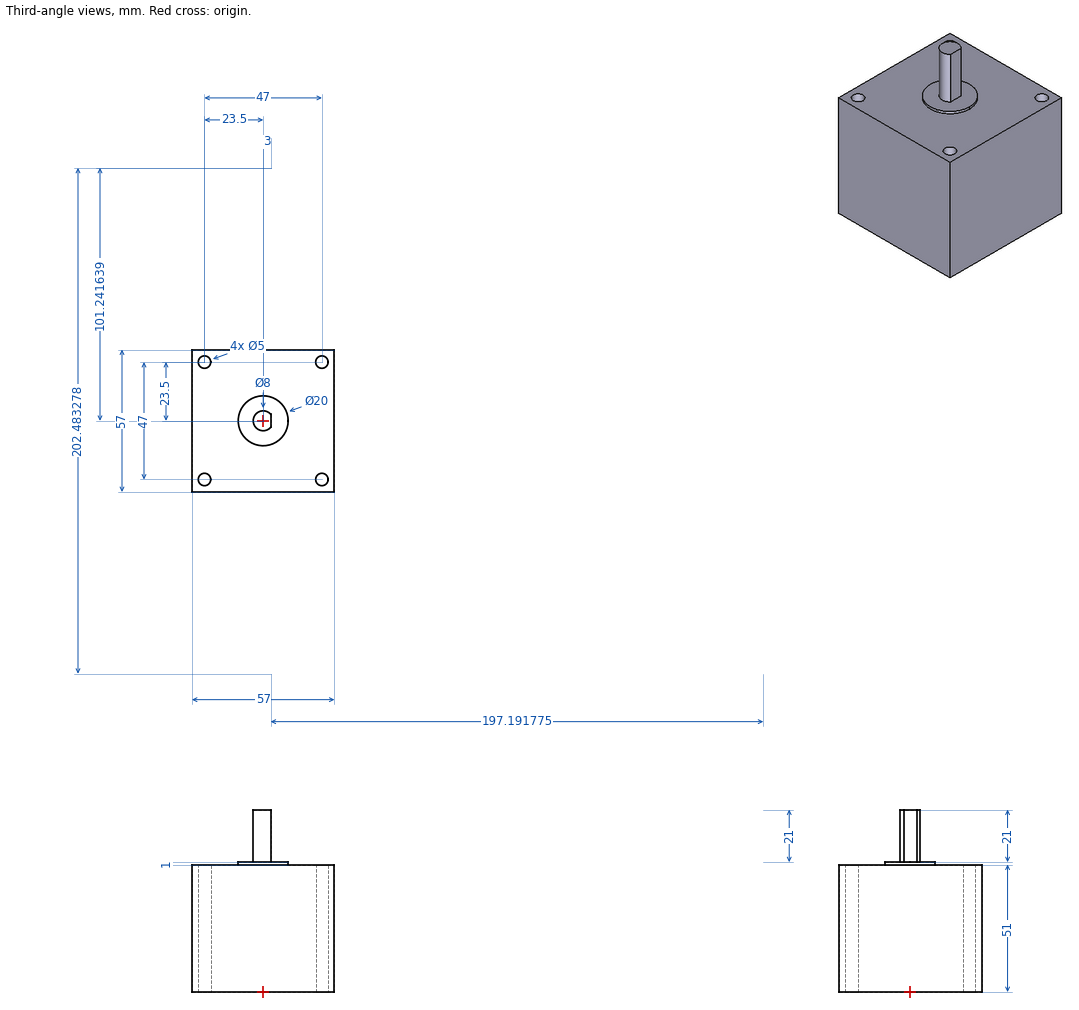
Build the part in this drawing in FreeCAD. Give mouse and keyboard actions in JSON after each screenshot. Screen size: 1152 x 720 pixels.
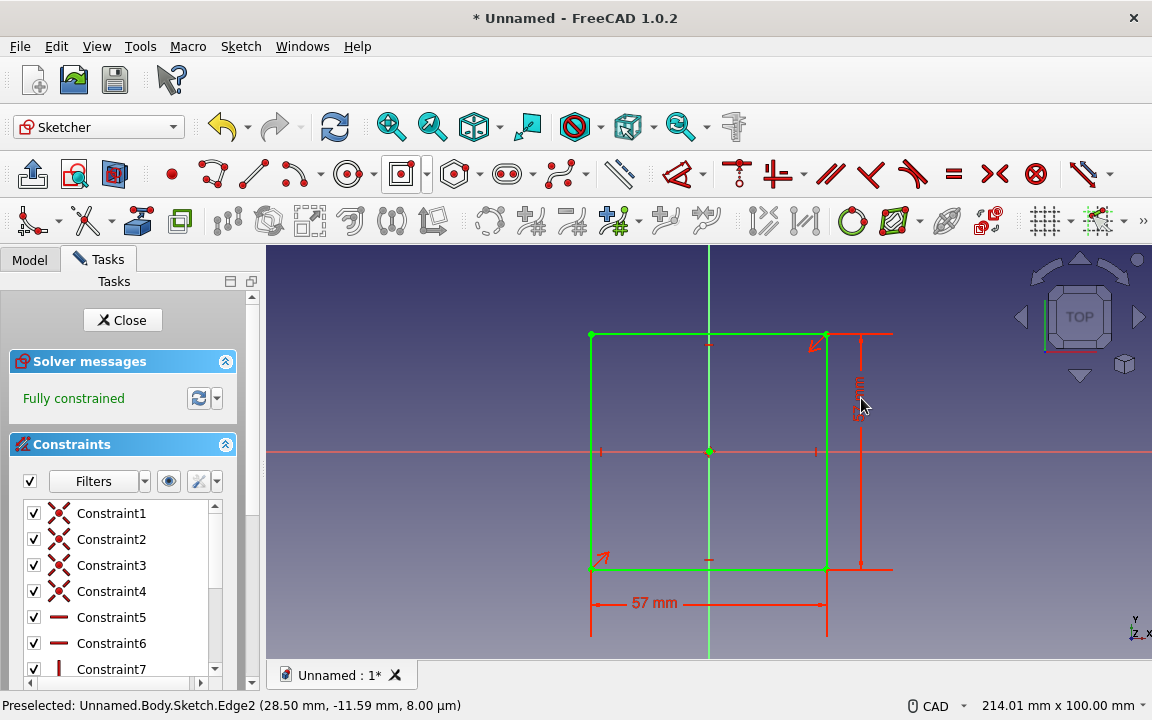
{"action": "left_click", "coordinate": [123, 320]}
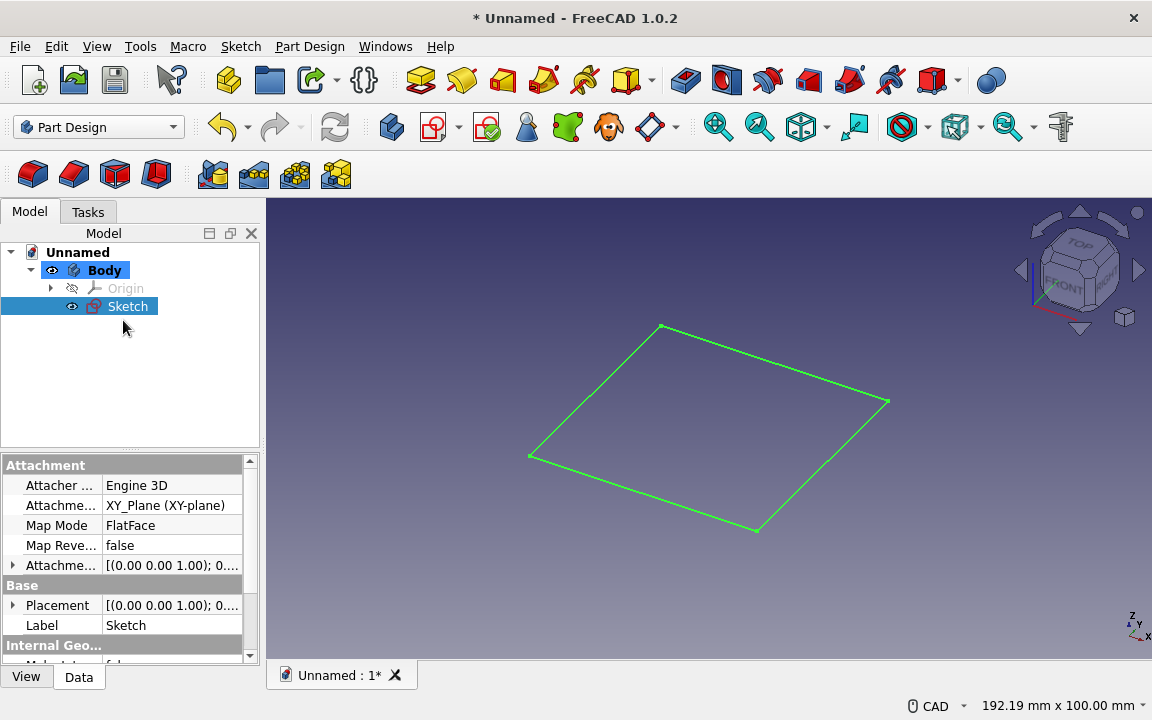
{"action": "left_click", "coordinate": [421, 80]}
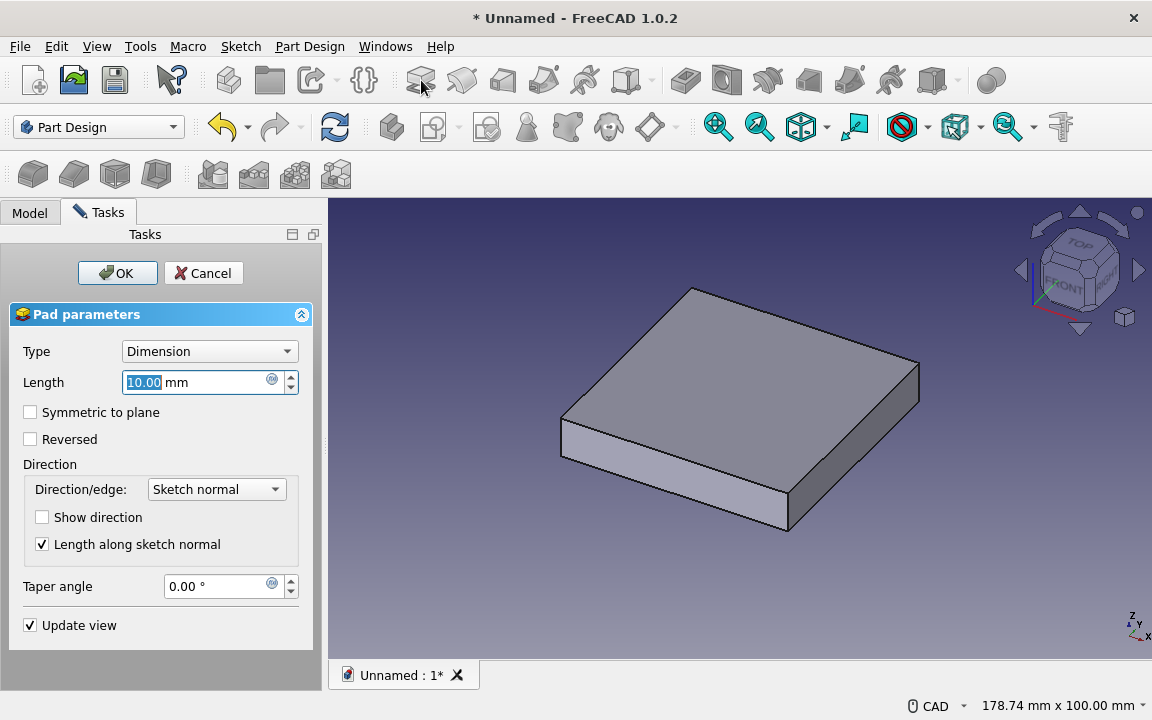
{"action": "type", "text": "51"}
{"action": "key", "text": "Tab"}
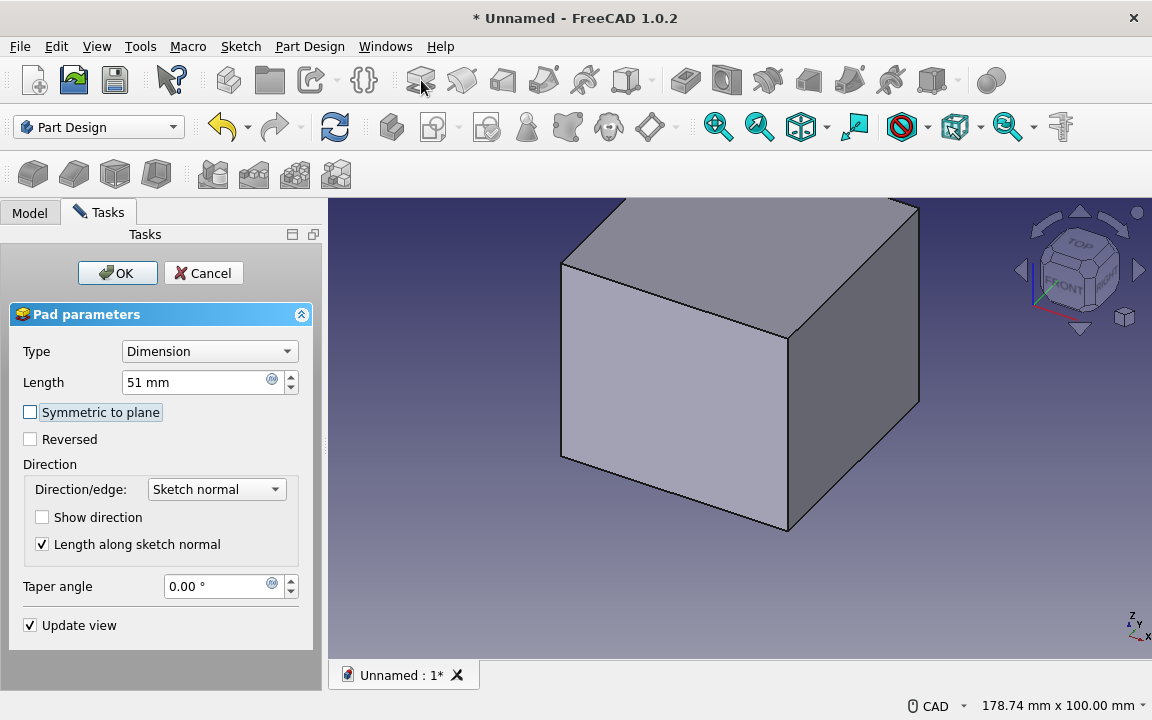
{"action": "left_click", "coordinate": [118, 273]}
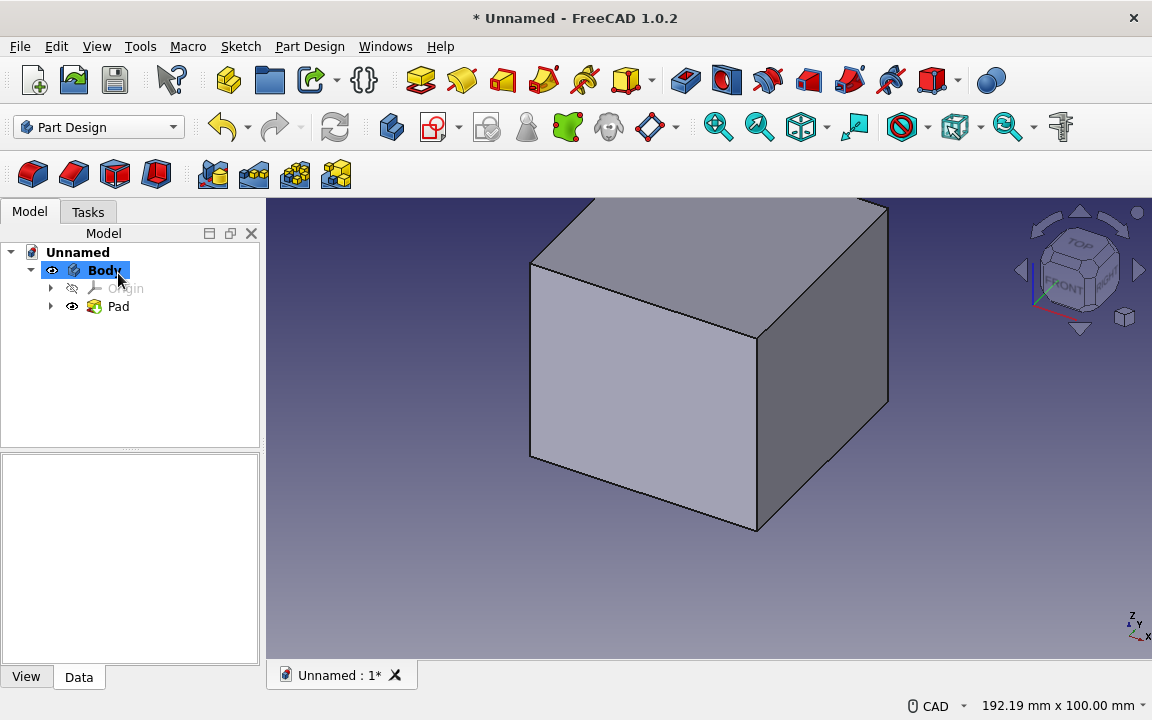
{"action": "left_click", "coordinate": [719, 128]}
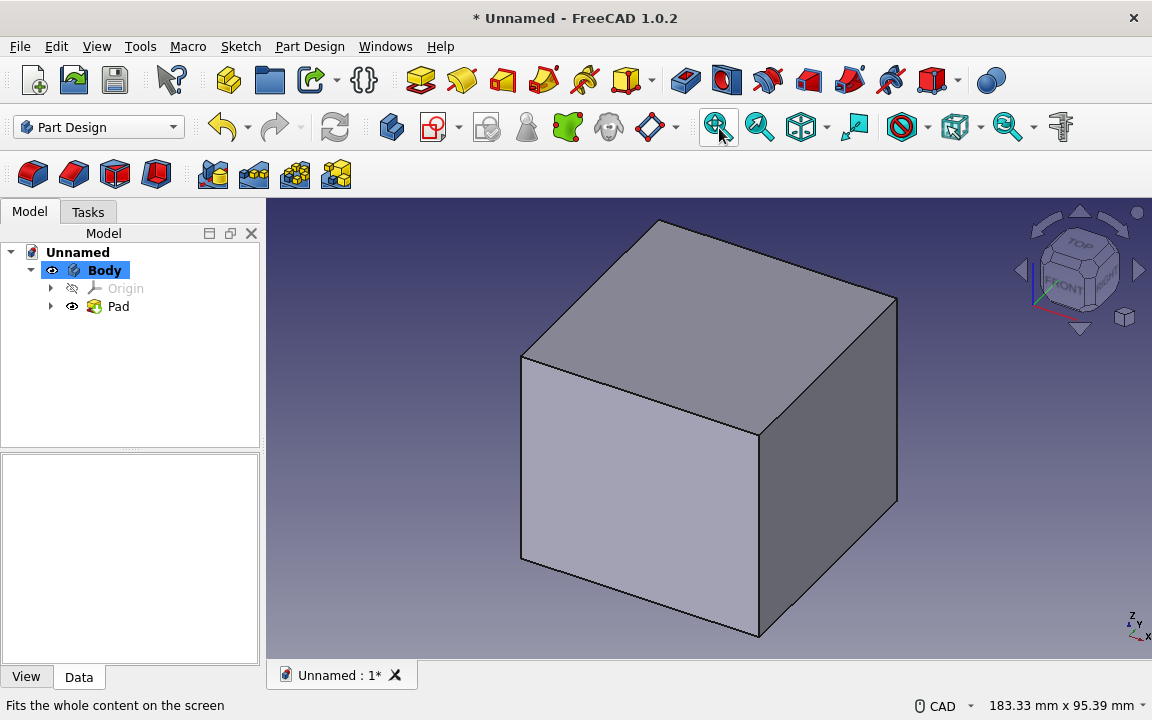
{"action": "left_click", "coordinate": [709, 327]}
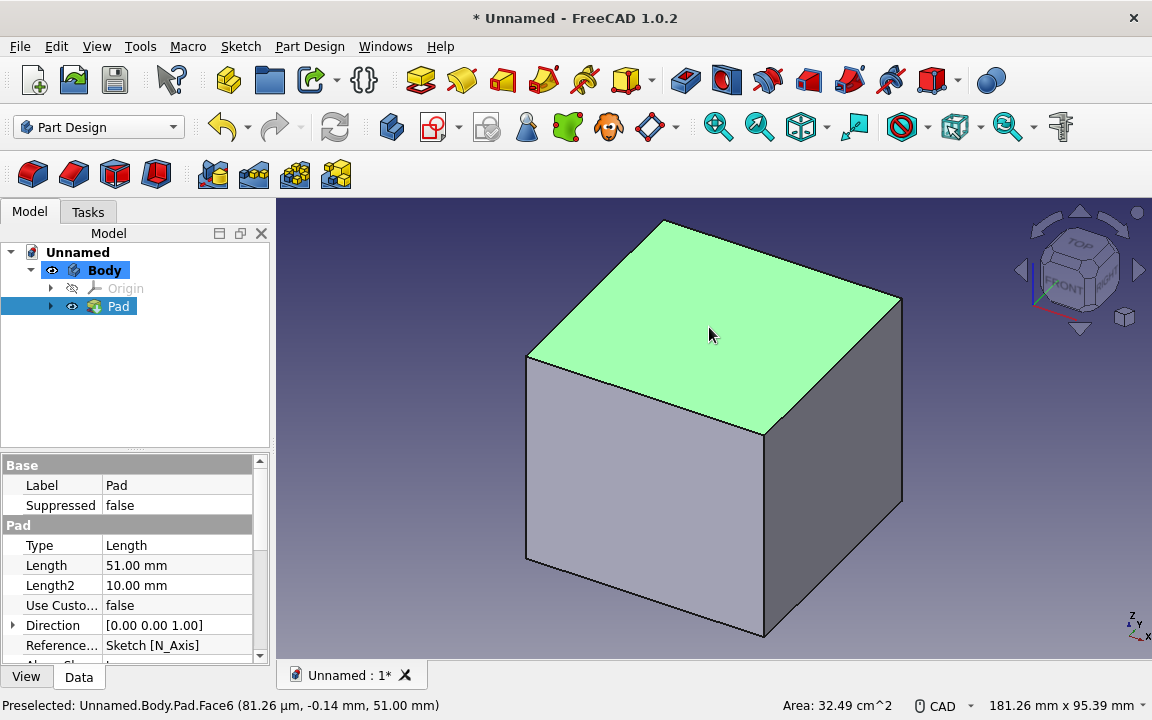
{"action": "left_click", "coordinate": [432, 128]}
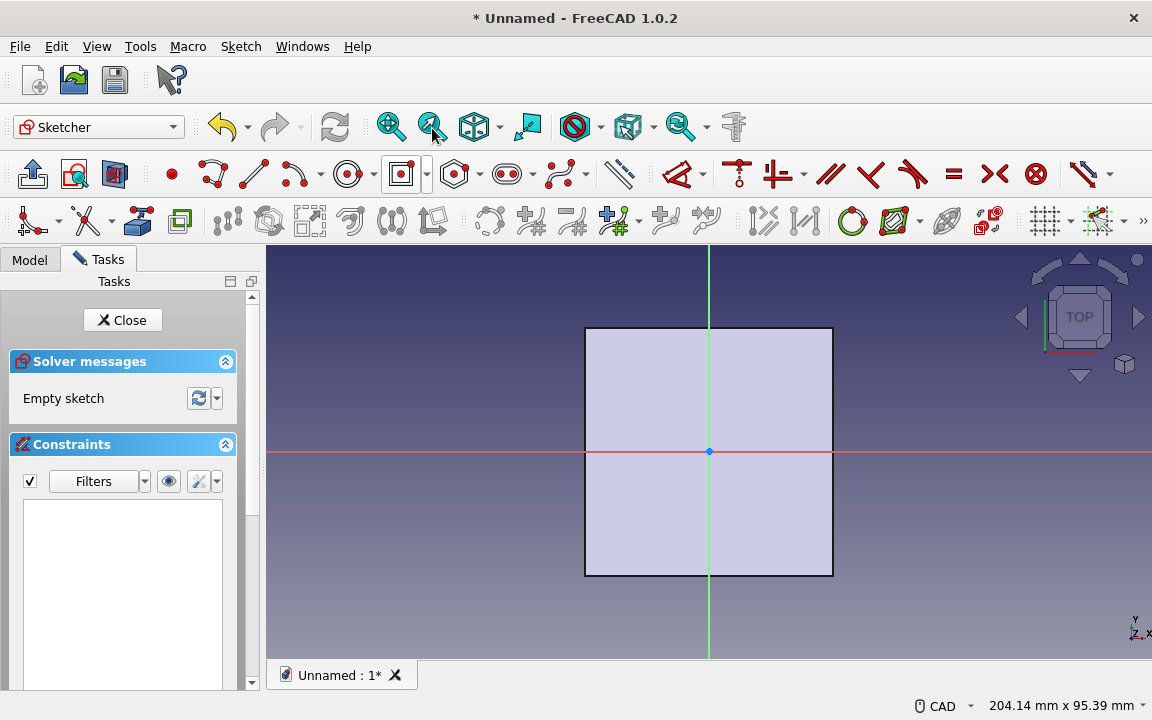
{"action": "left_click", "coordinate": [348, 174]}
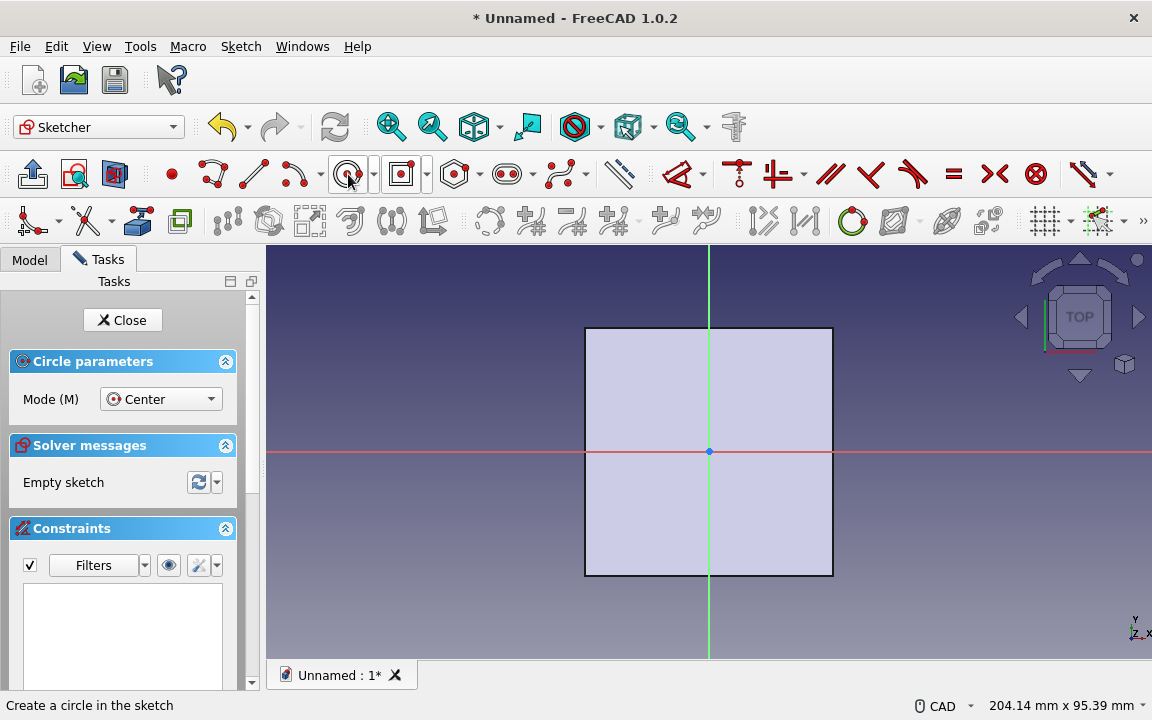
{"action": "scroll", "coordinate": [607, 350], "scroll_direction": "up", "scroll_amount": 4}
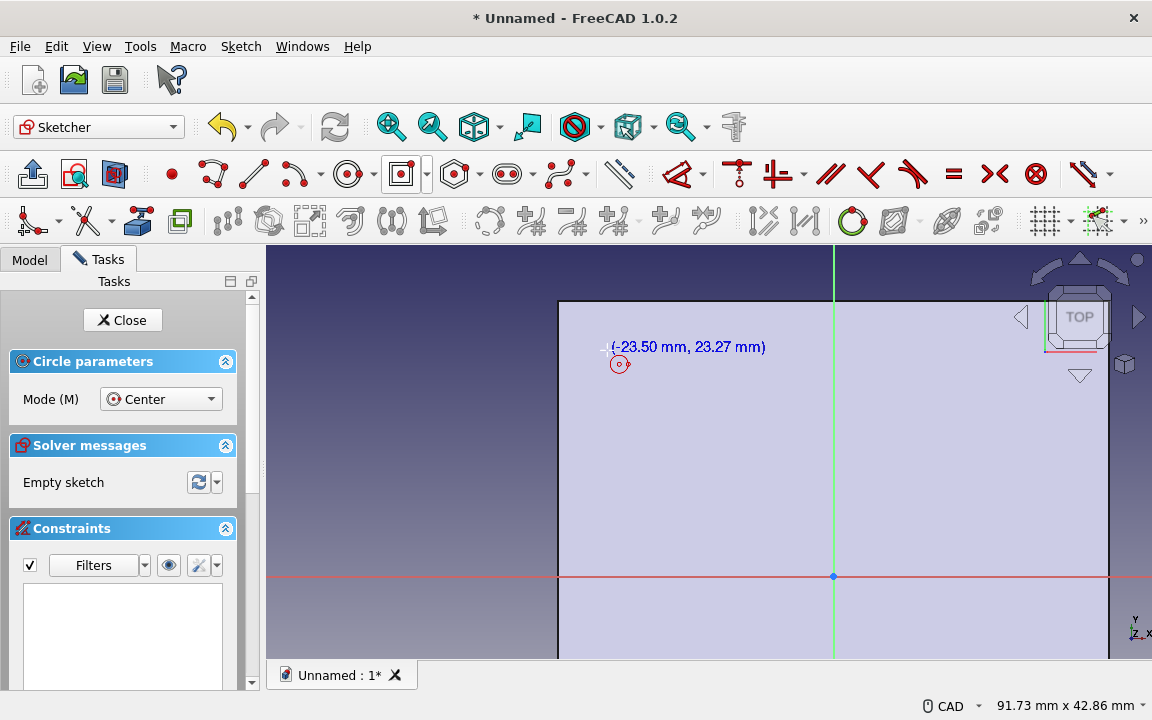
{"action": "left_click", "coordinate": [607, 350]}
{"action": "left_click", "coordinate": [624, 333]}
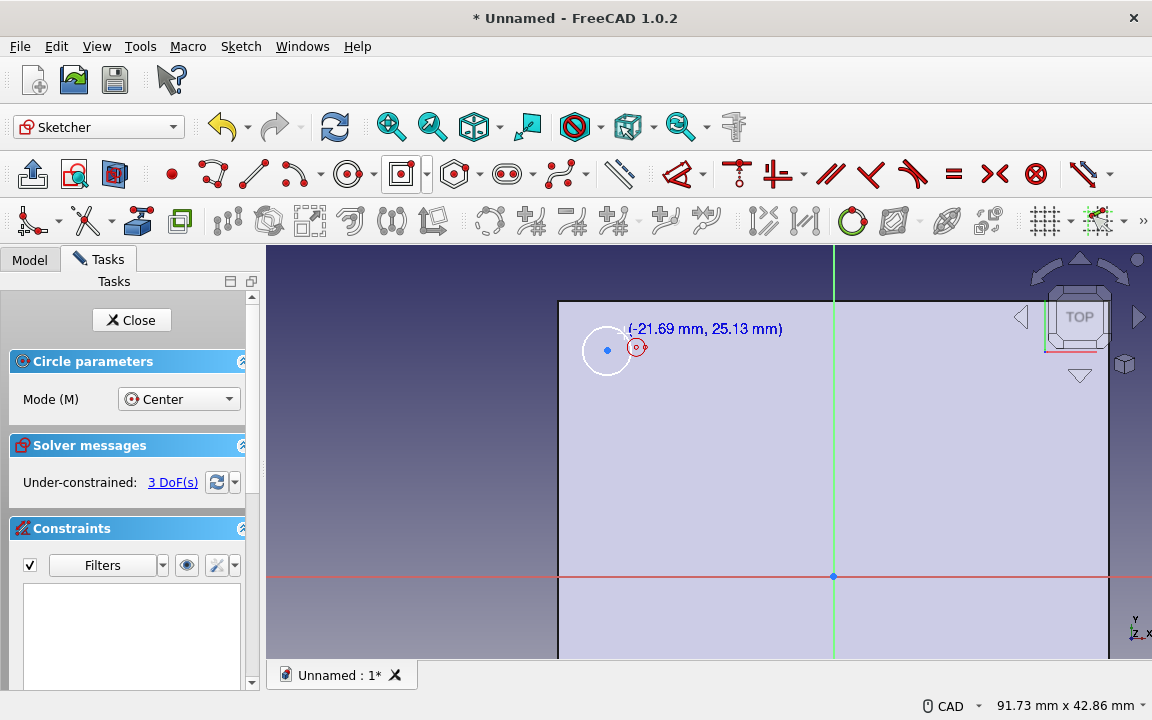
{"action": "scroll", "coordinate": [406, 300], "scroll_direction": "down", "scroll_amount": 3}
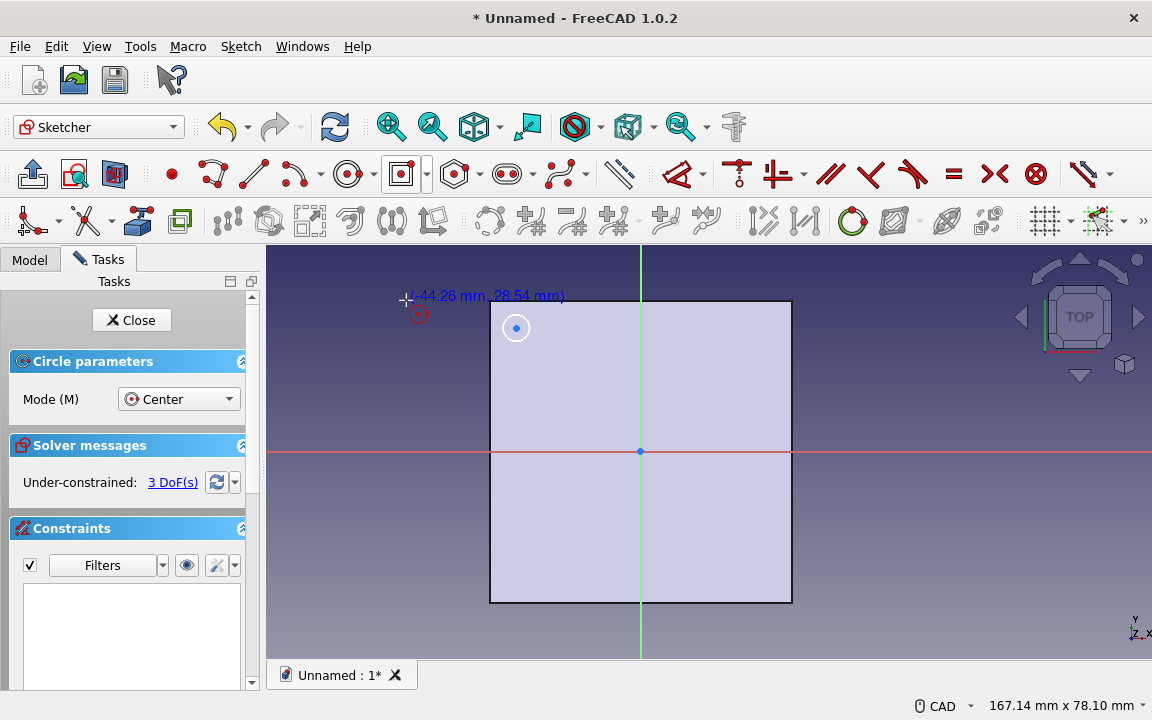
{"action": "scroll", "coordinate": [765, 327], "scroll_direction": "up", "scroll_amount": 3}